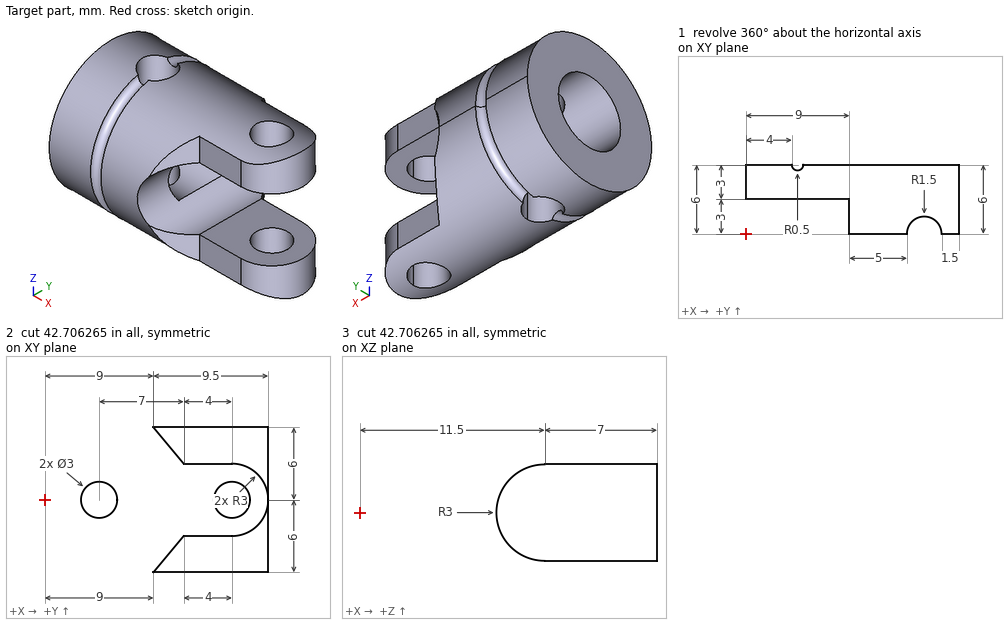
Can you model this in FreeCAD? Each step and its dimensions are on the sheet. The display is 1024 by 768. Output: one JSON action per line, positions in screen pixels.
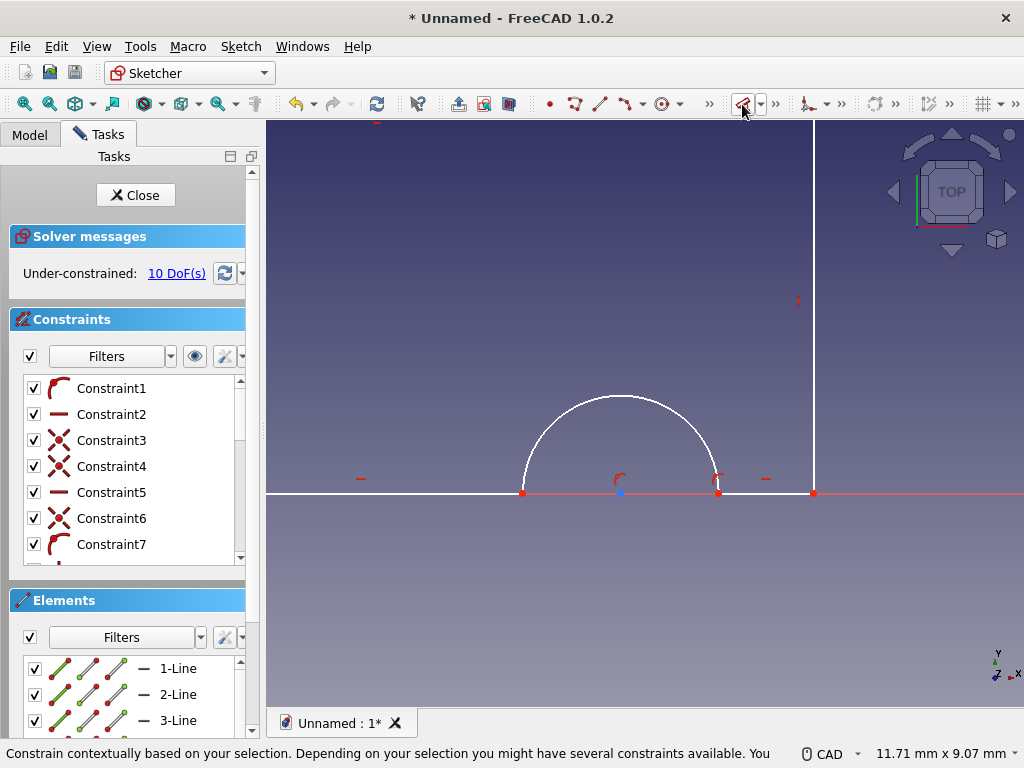
{"action": "left_click", "coordinate": [678, 414]}
{"action": "left_click", "coordinate": [697, 388]}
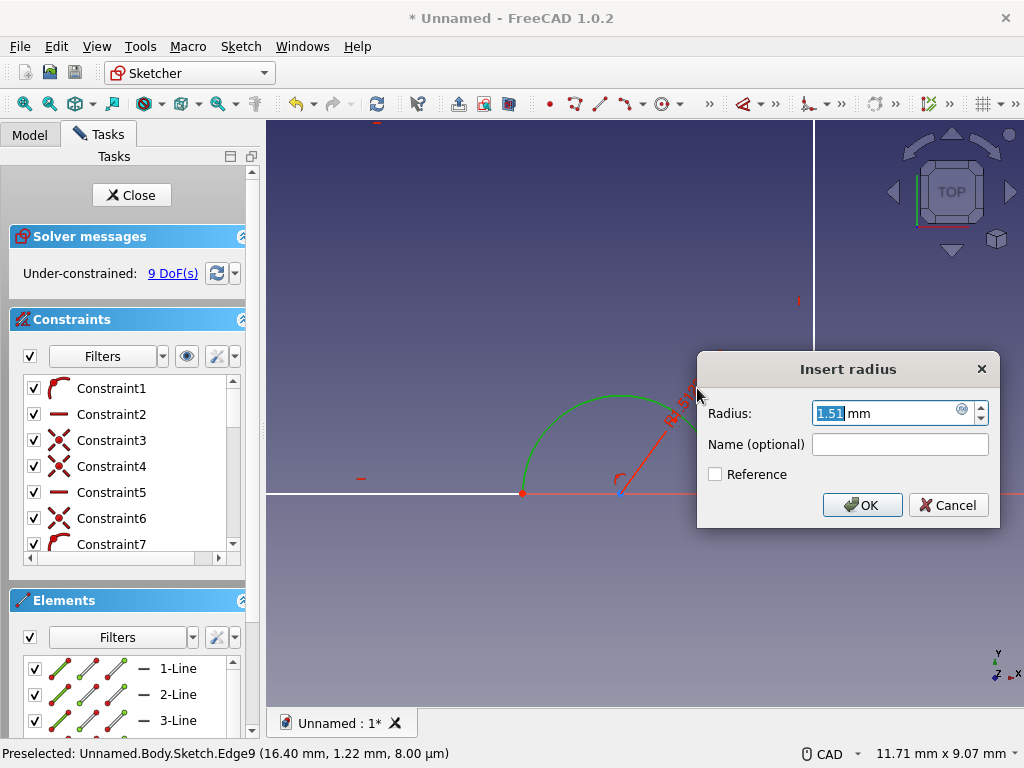
{"action": "type", "text": "1.5"}
{"action": "key", "text": "Return"}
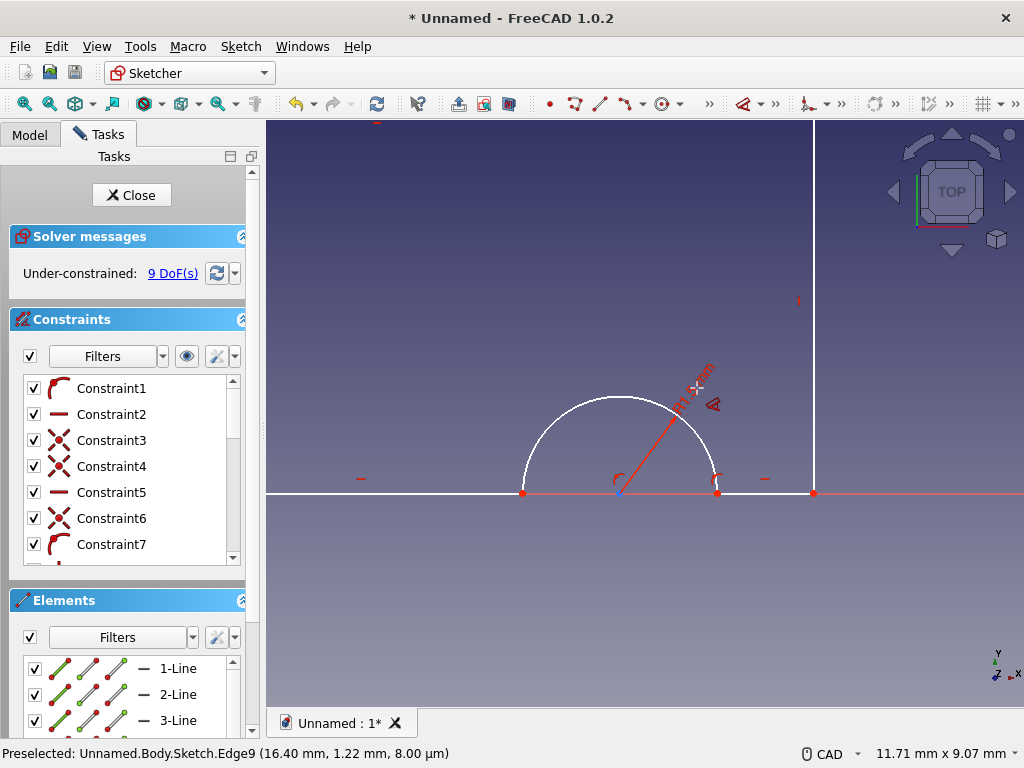
{"action": "scroll", "coordinate": [786, 480], "scroll_direction": "down", "scroll_amount": 5}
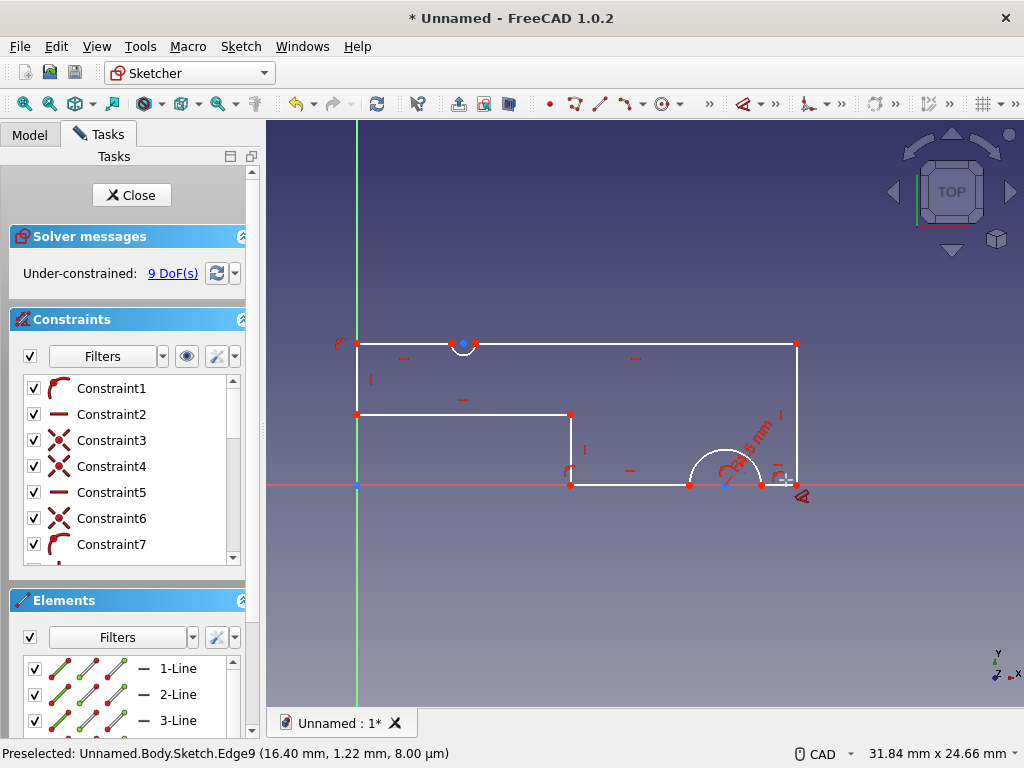
{"action": "scroll", "coordinate": [457, 353], "scroll_direction": "up", "scroll_amount": 7}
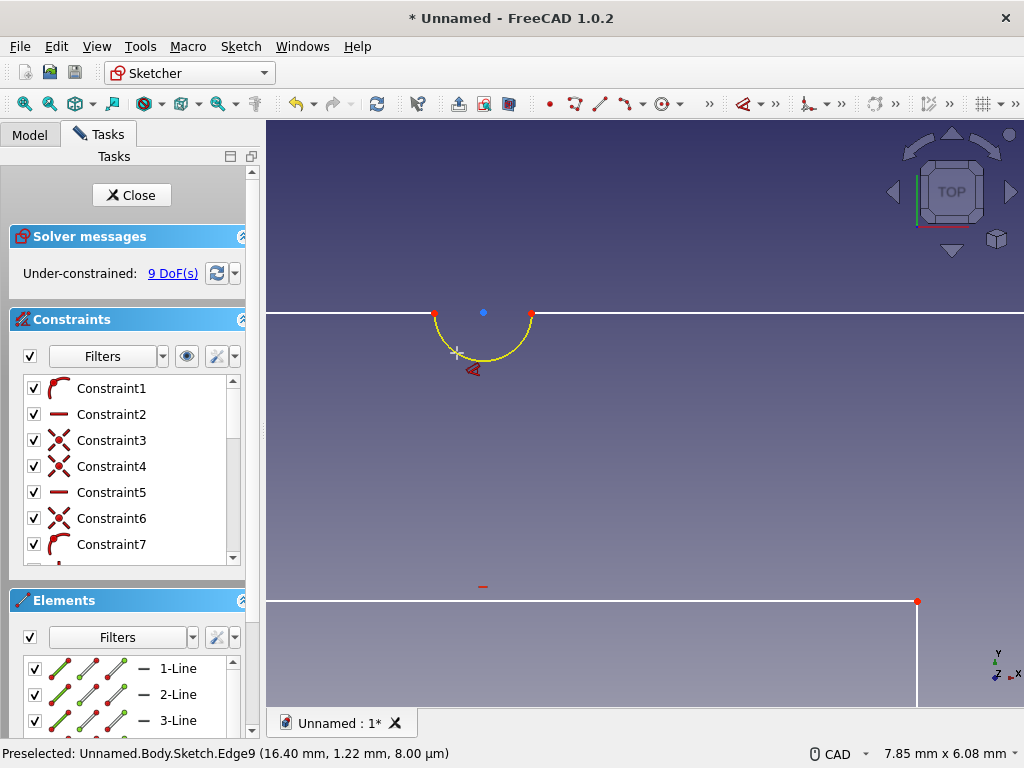
{"action": "left_click", "coordinate": [455, 352]}
{"action": "left_click", "coordinate": [436, 378]}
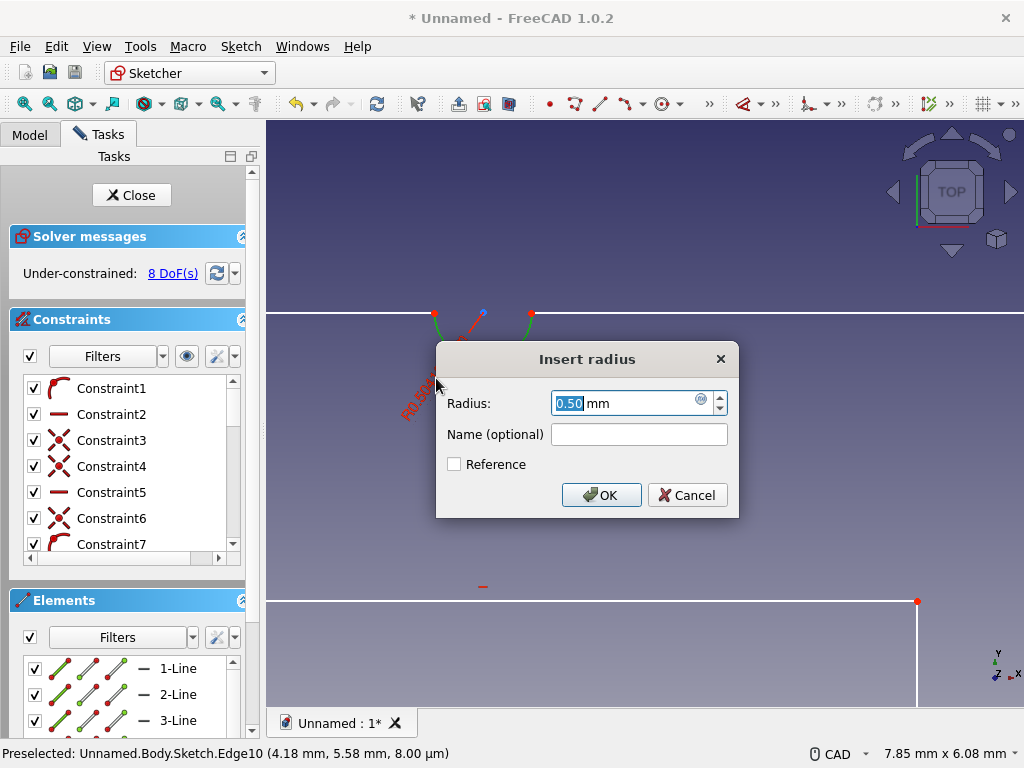
{"action": "type", "text": "0.5"}
{"action": "key", "text": "Return"}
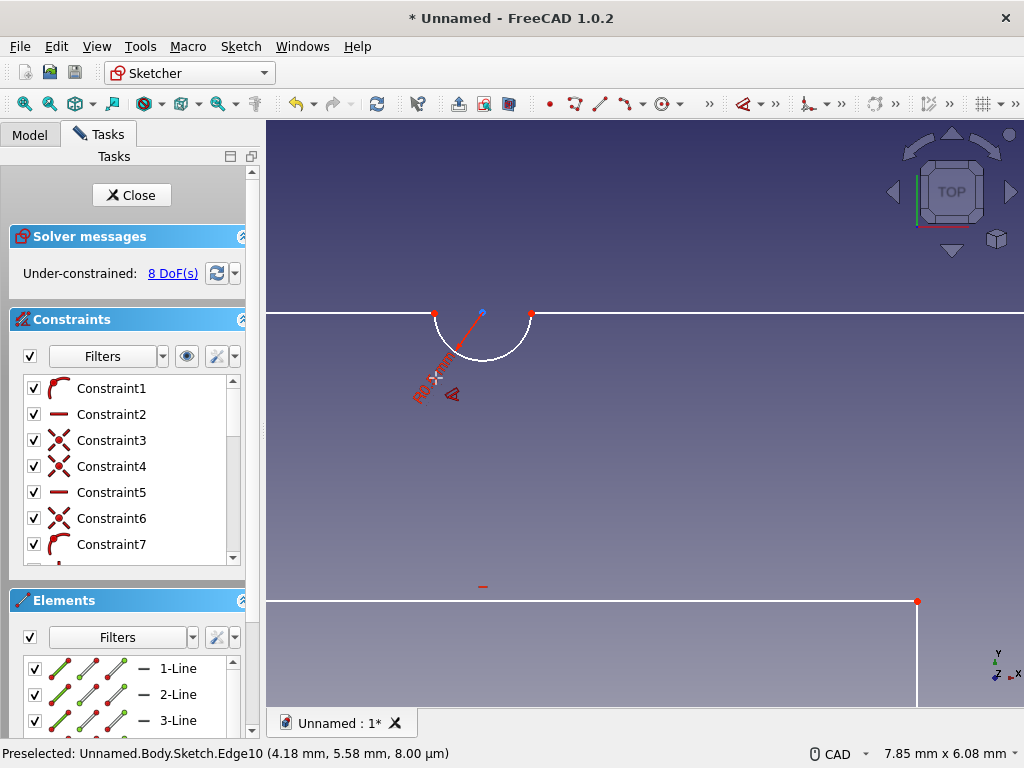
{"action": "scroll", "coordinate": [457, 353], "scroll_direction": "down", "scroll_amount": 7}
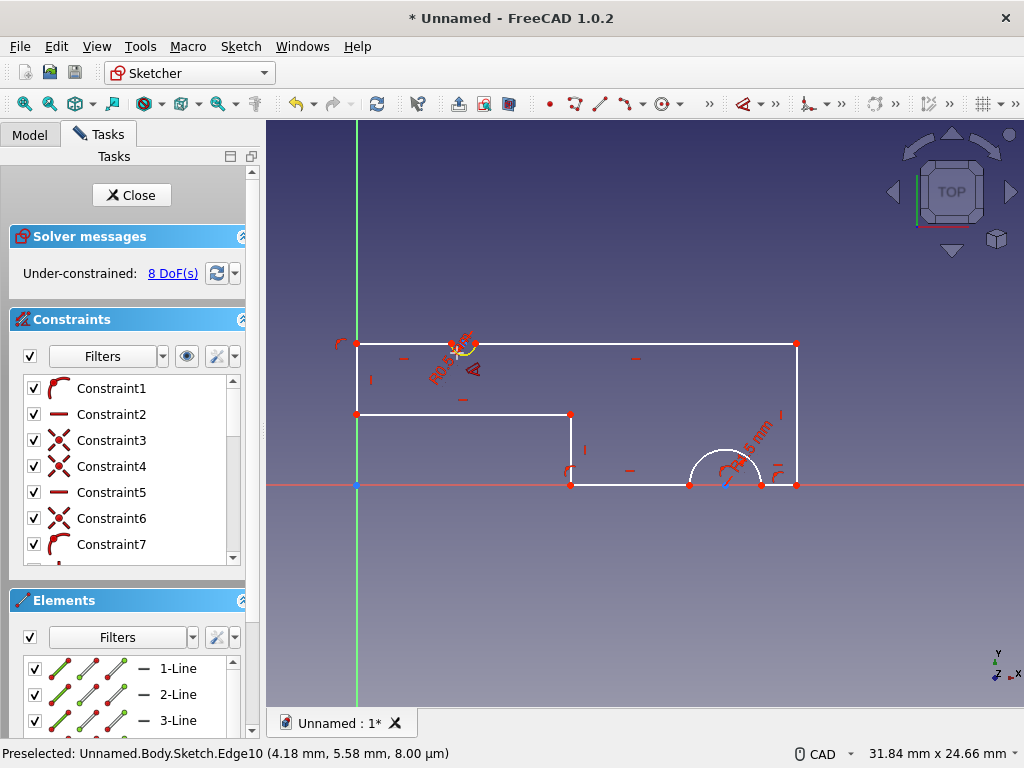
{"action": "left_click", "coordinate": [423, 344]}
{"action": "left_click", "coordinate": [404, 310]}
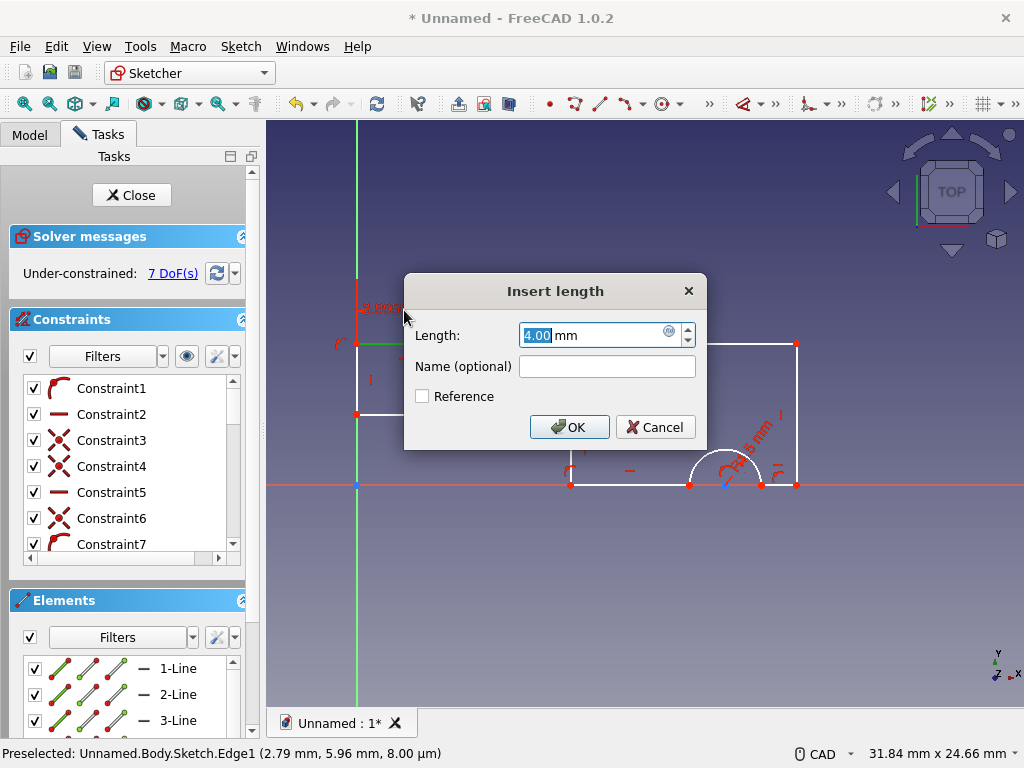
{"action": "type", "text": "4"}
{"action": "key", "text": "Return"}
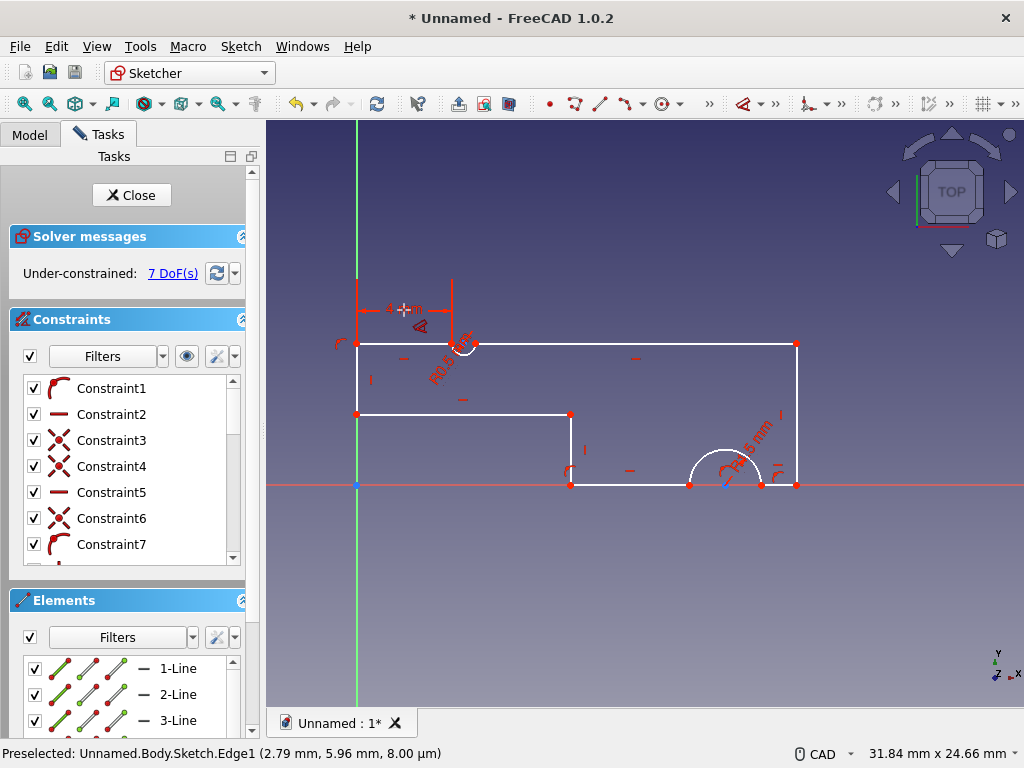
{"action": "left_click", "coordinate": [357, 365]}
{"action": "left_click", "coordinate": [323, 379]}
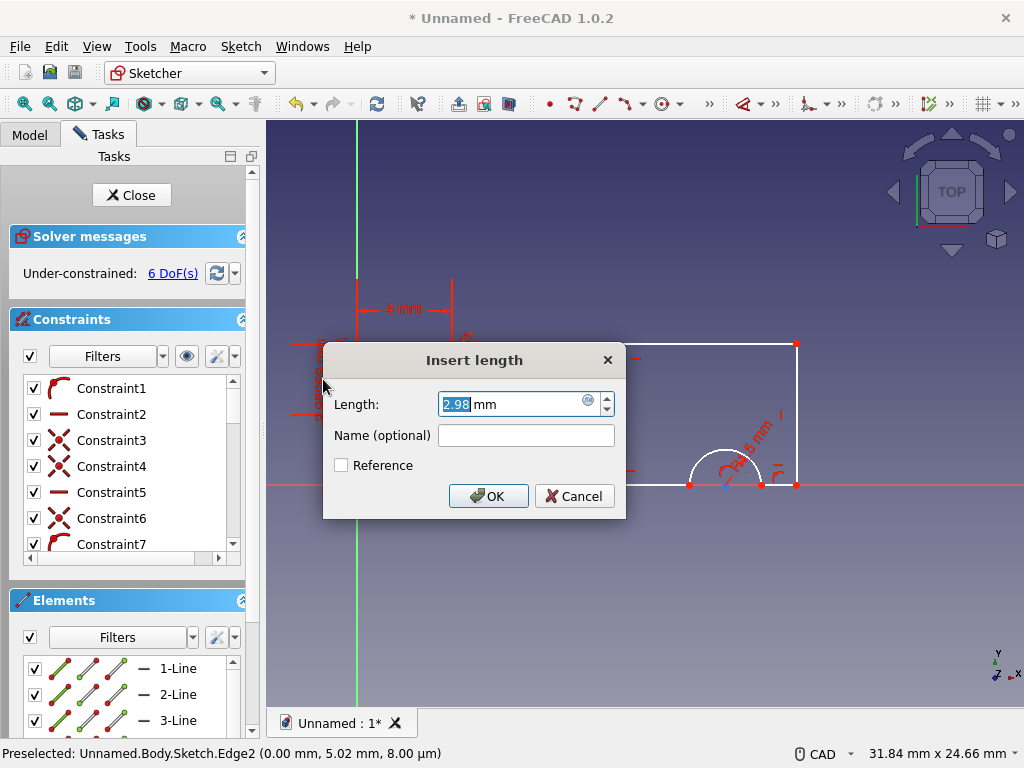
{"action": "type", "text": "3"}
{"action": "key", "text": "Return"}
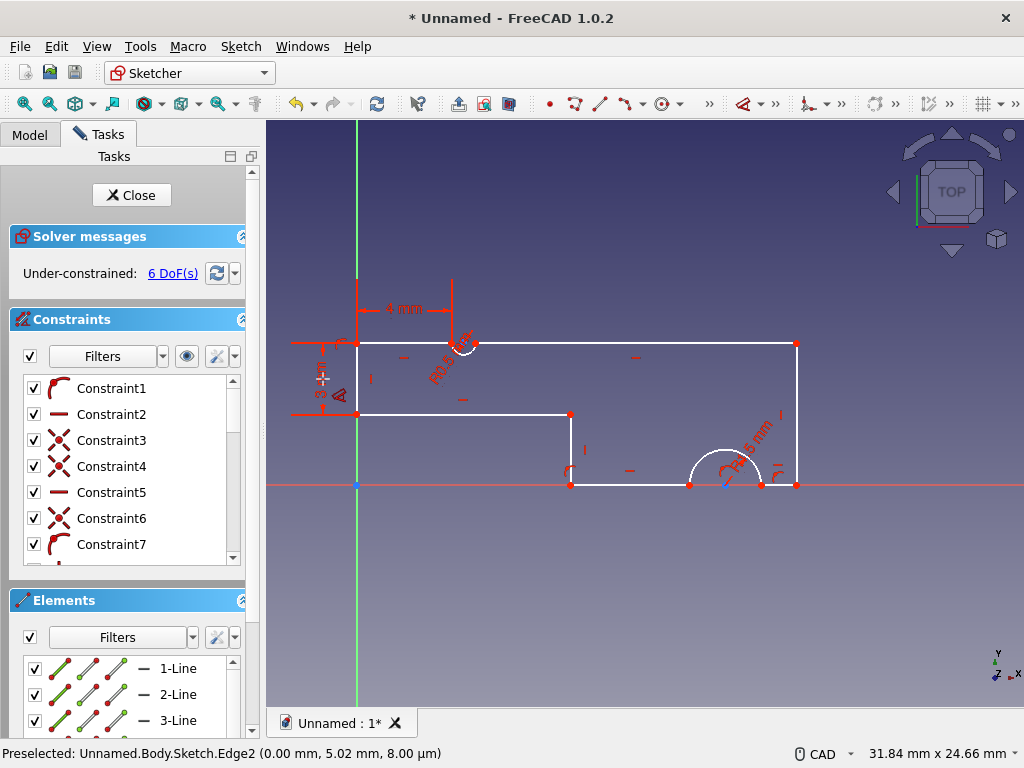
{"action": "left_click", "coordinate": [421, 415]}
{"action": "left_click", "coordinate": [464, 449]}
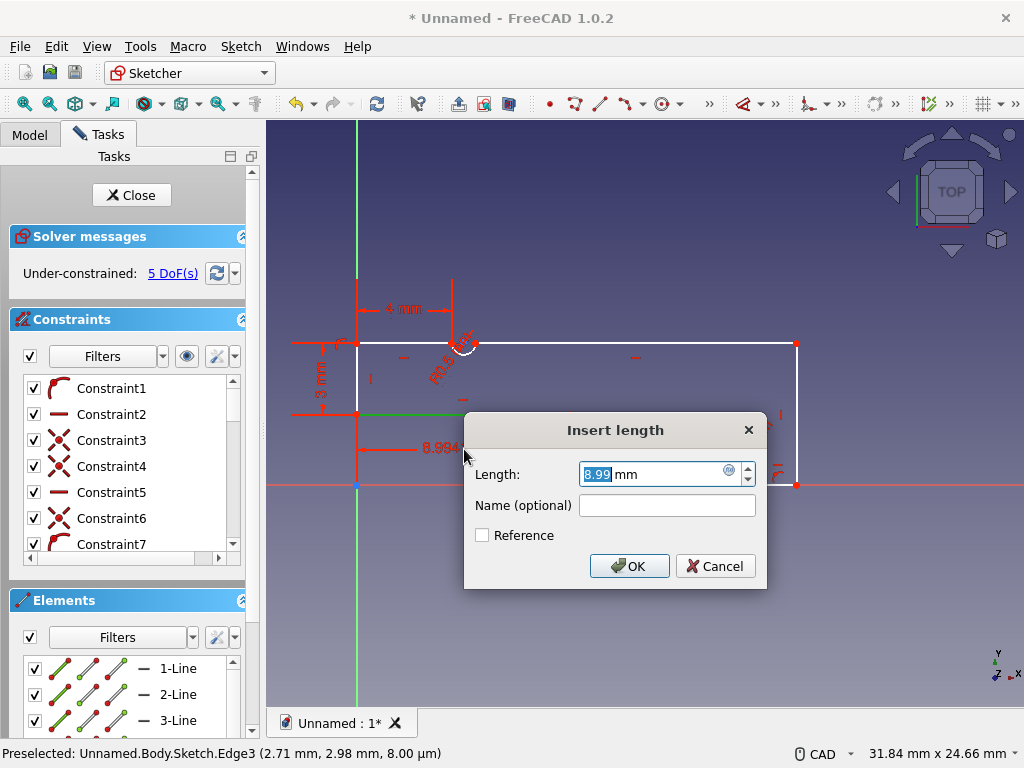
{"action": "type", "text": "9"}
{"action": "key", "text": "Return"}